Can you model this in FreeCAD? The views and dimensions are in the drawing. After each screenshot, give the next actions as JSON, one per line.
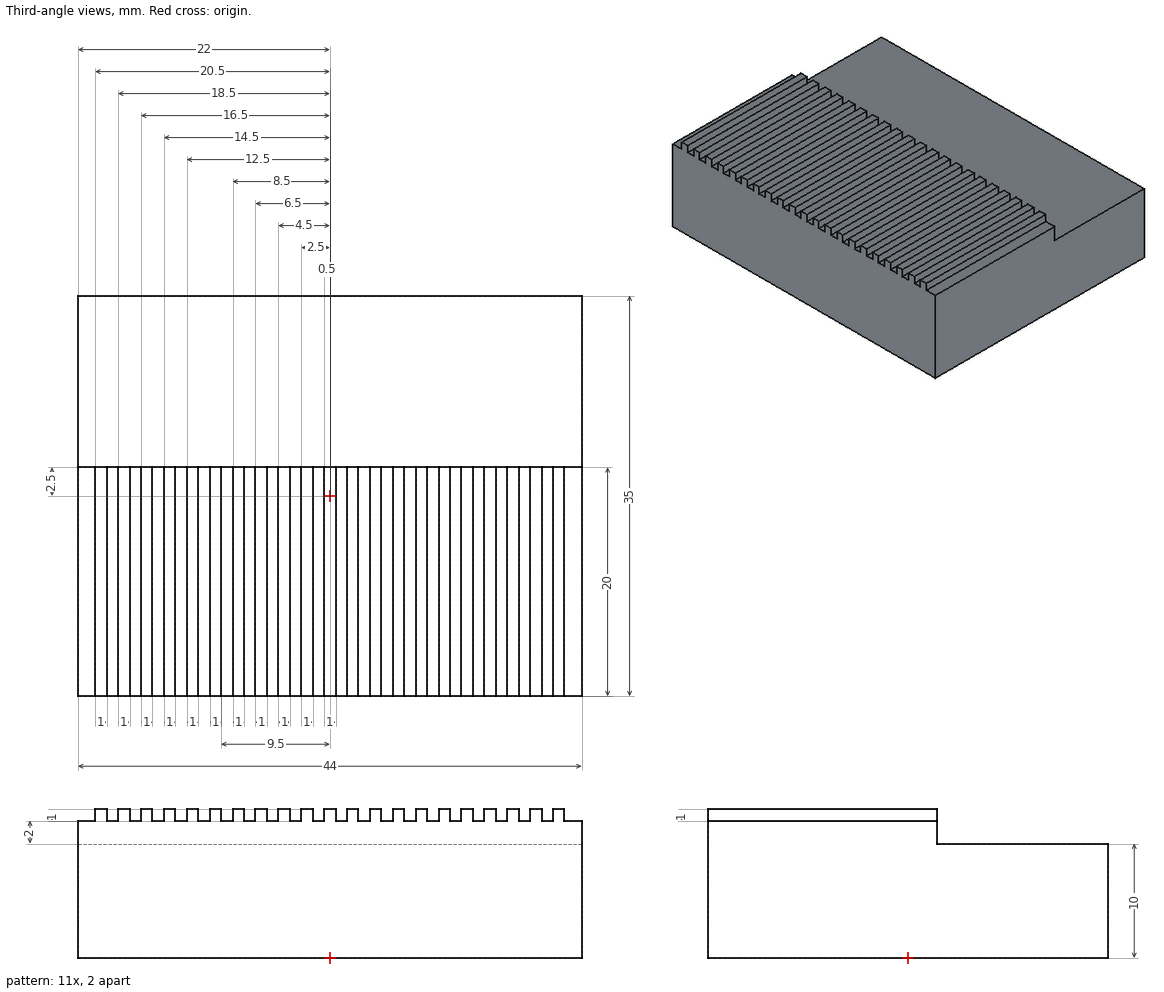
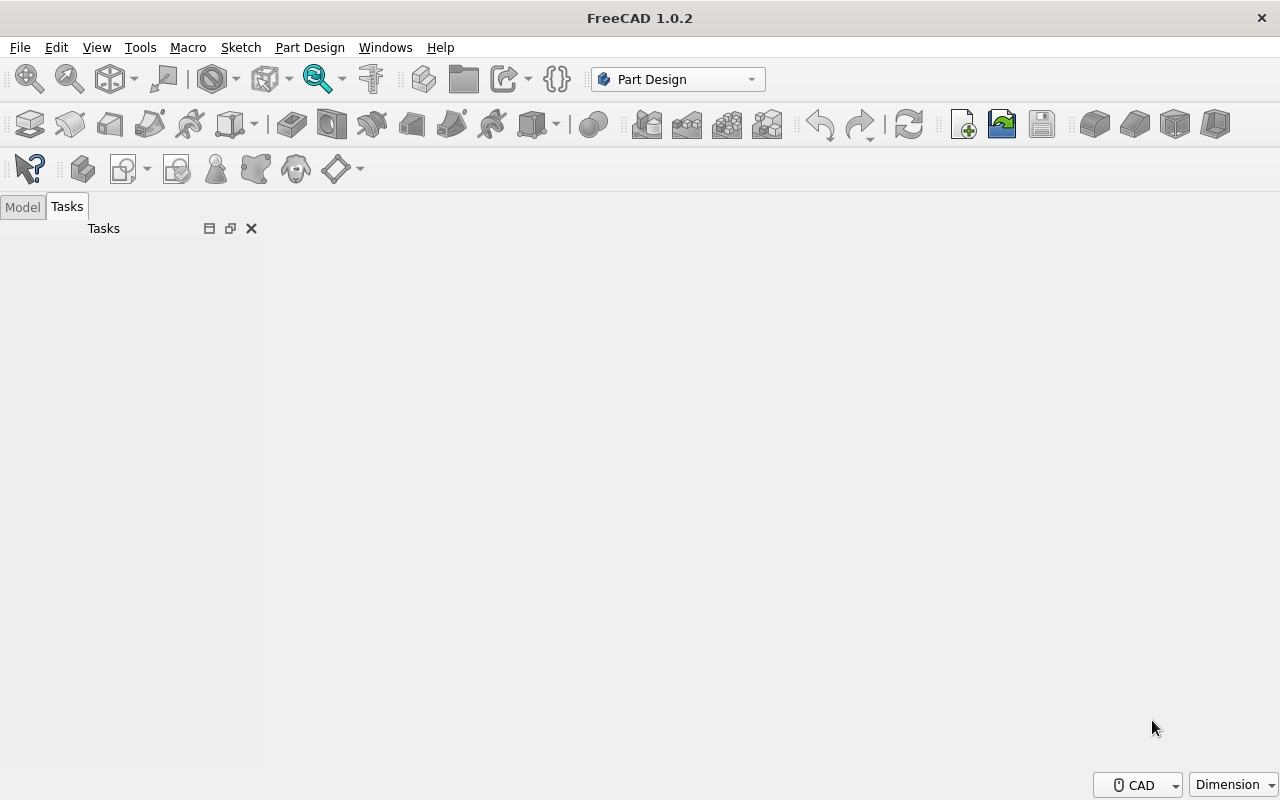
{"action": "left_click", "coordinate": [962, 124]}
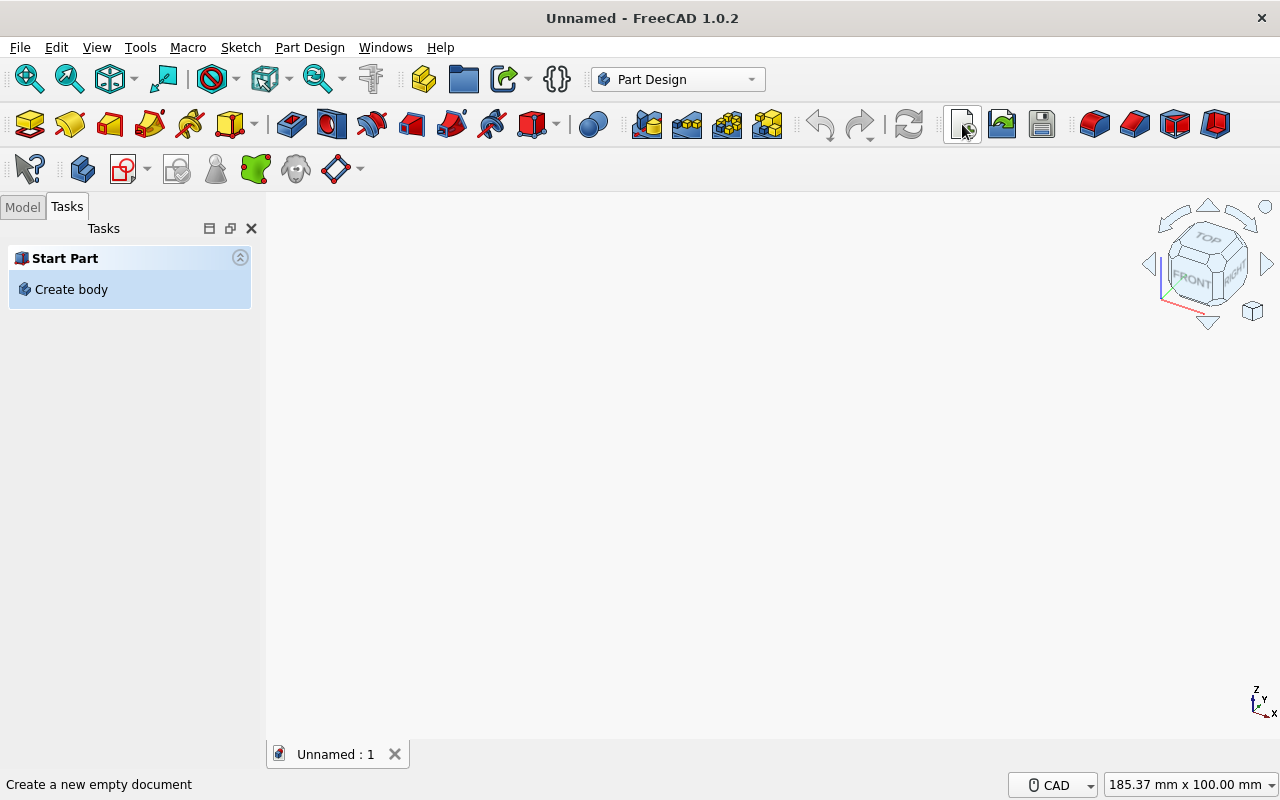
{"action": "left_click", "coordinate": [124, 170]}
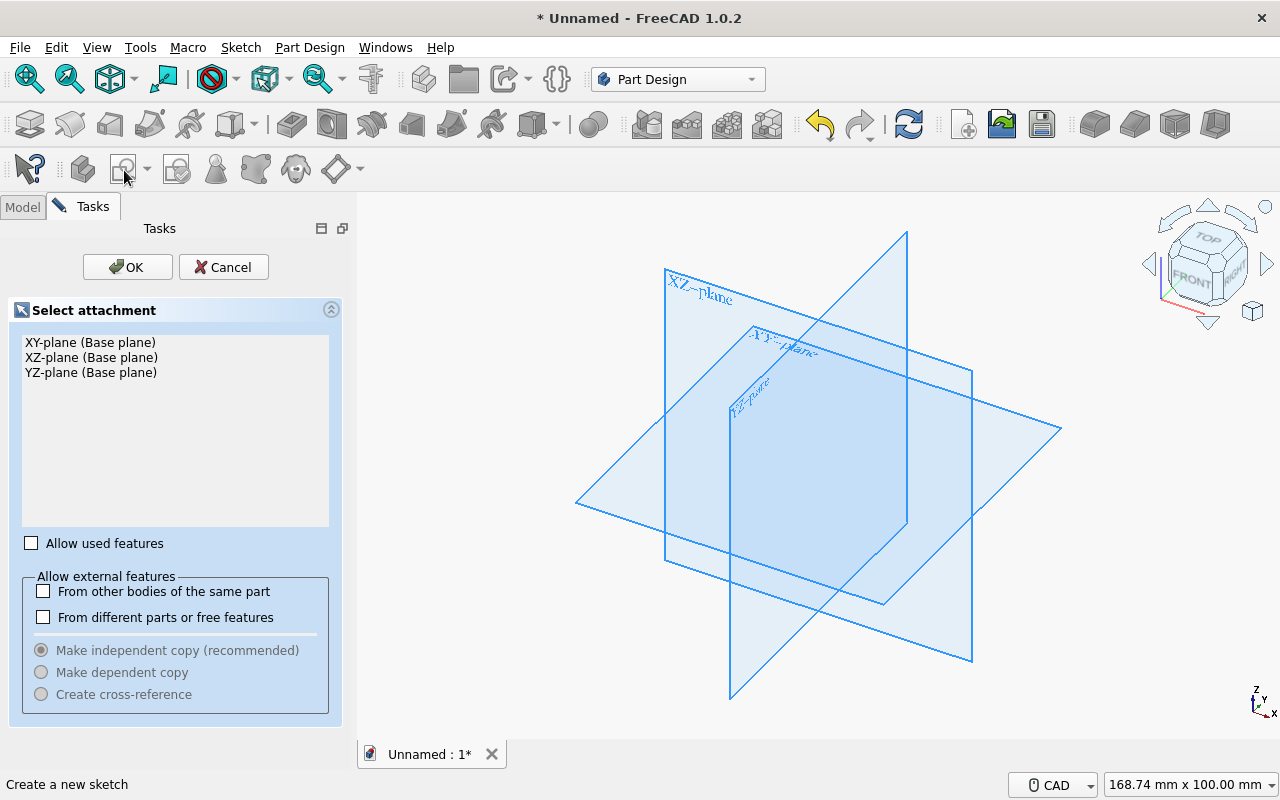
{"action": "left_click", "coordinate": [82, 342]}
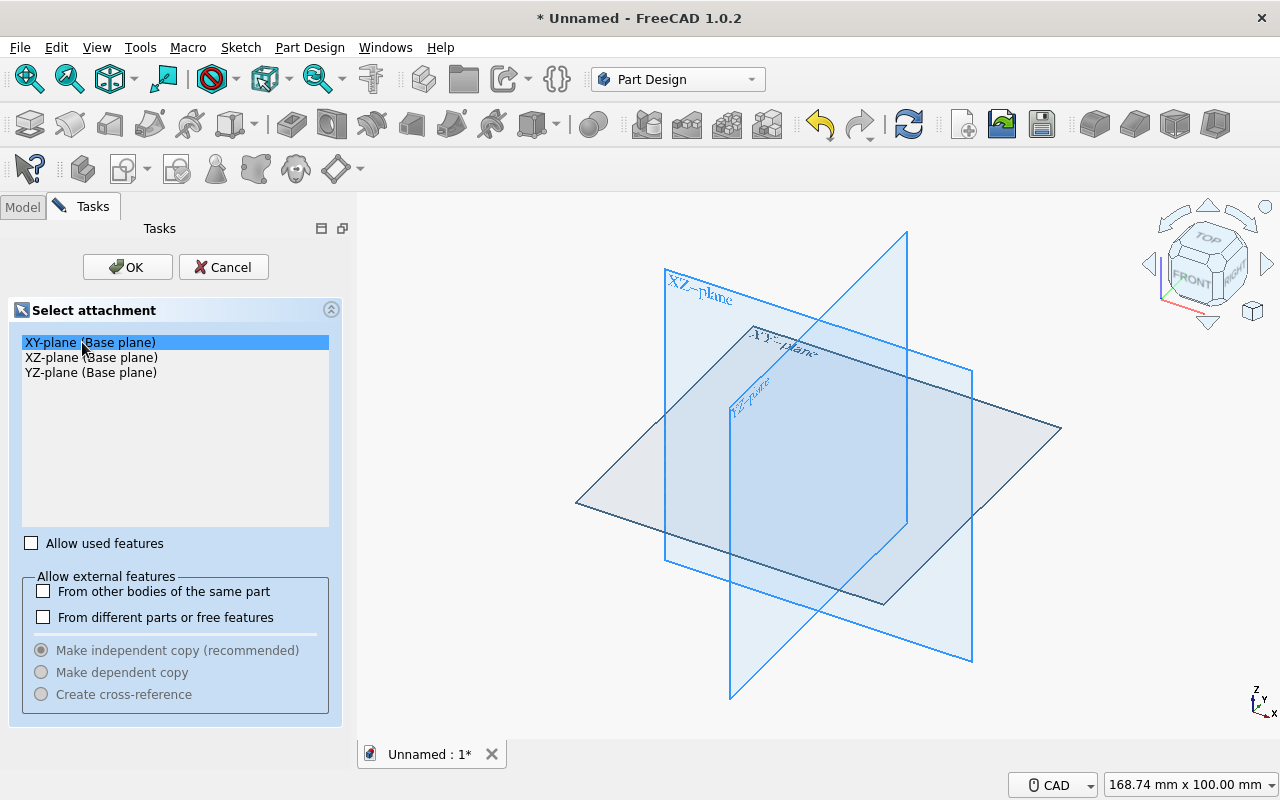
{"action": "left_click", "coordinate": [128, 267]}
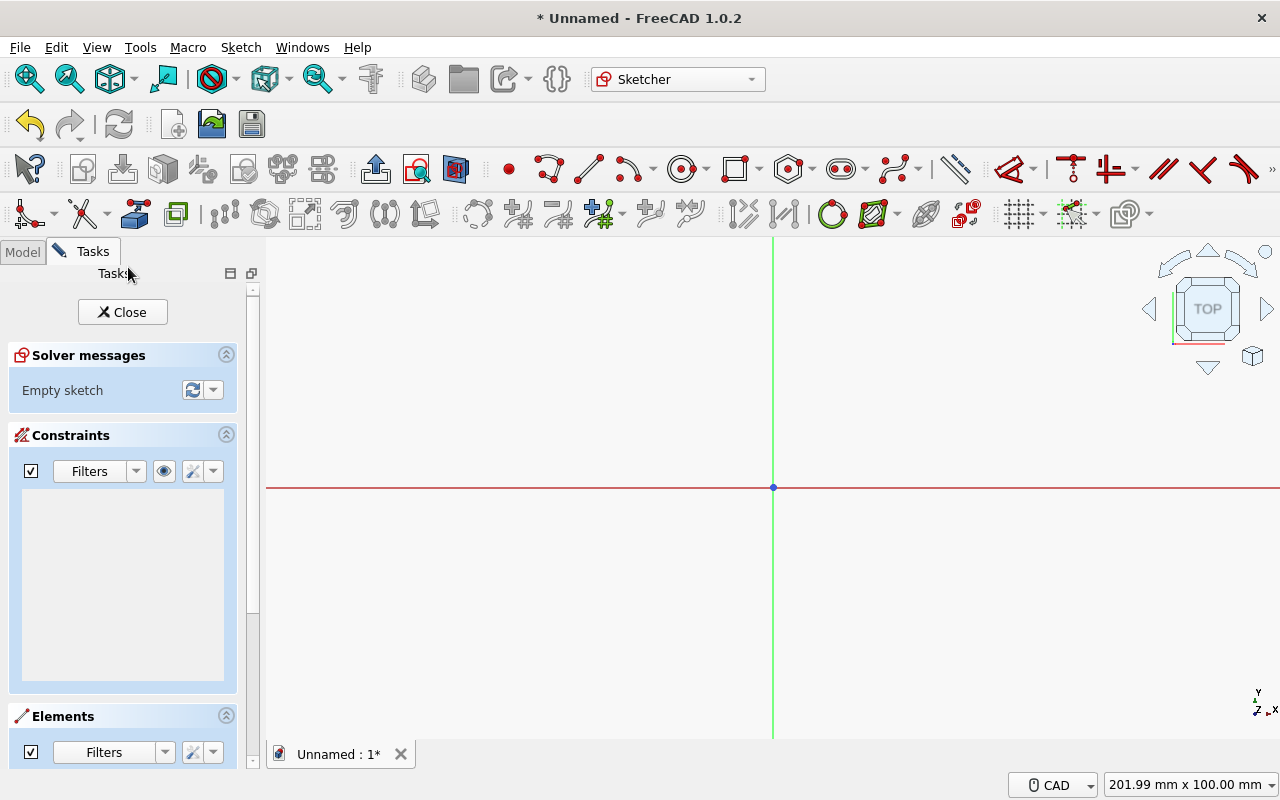
{"action": "scroll", "coordinate": [856, 488], "scroll_direction": "up", "scroll_amount": 3}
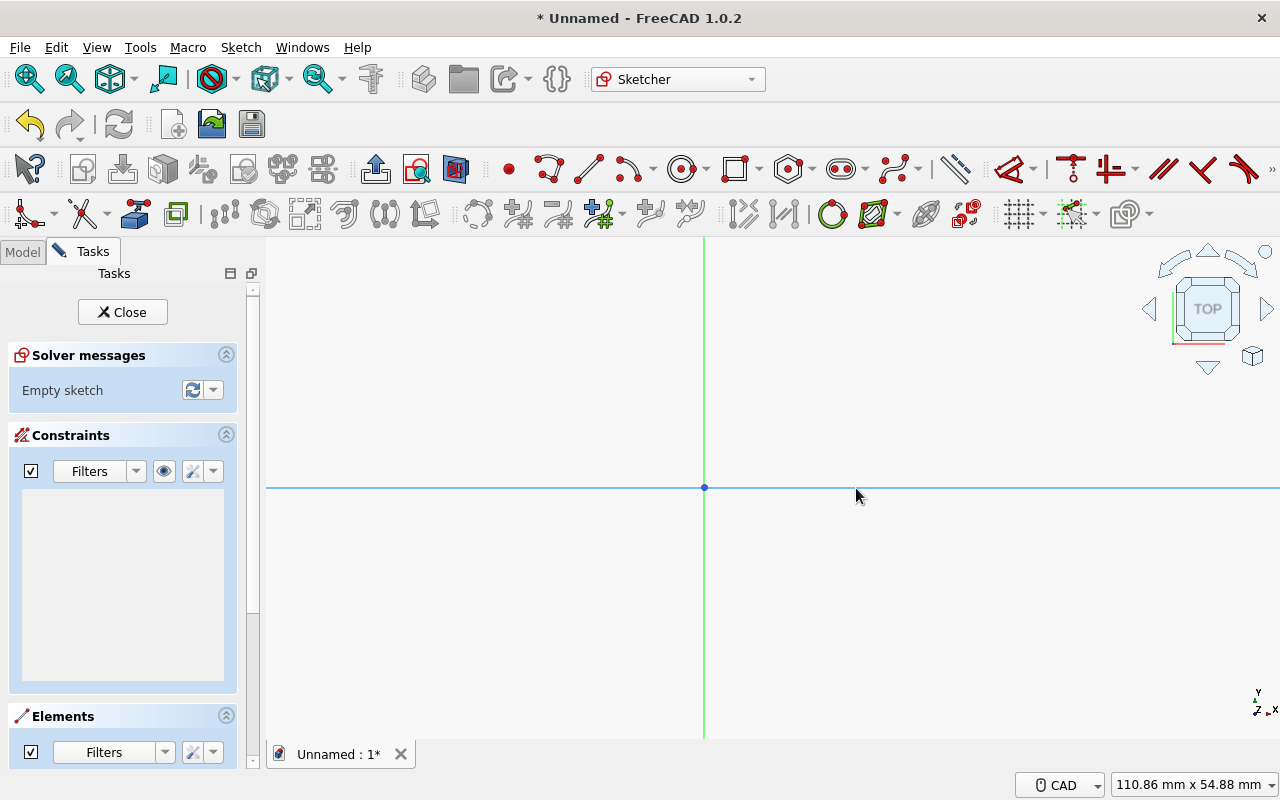
{"action": "left_click", "coordinate": [762, 170]}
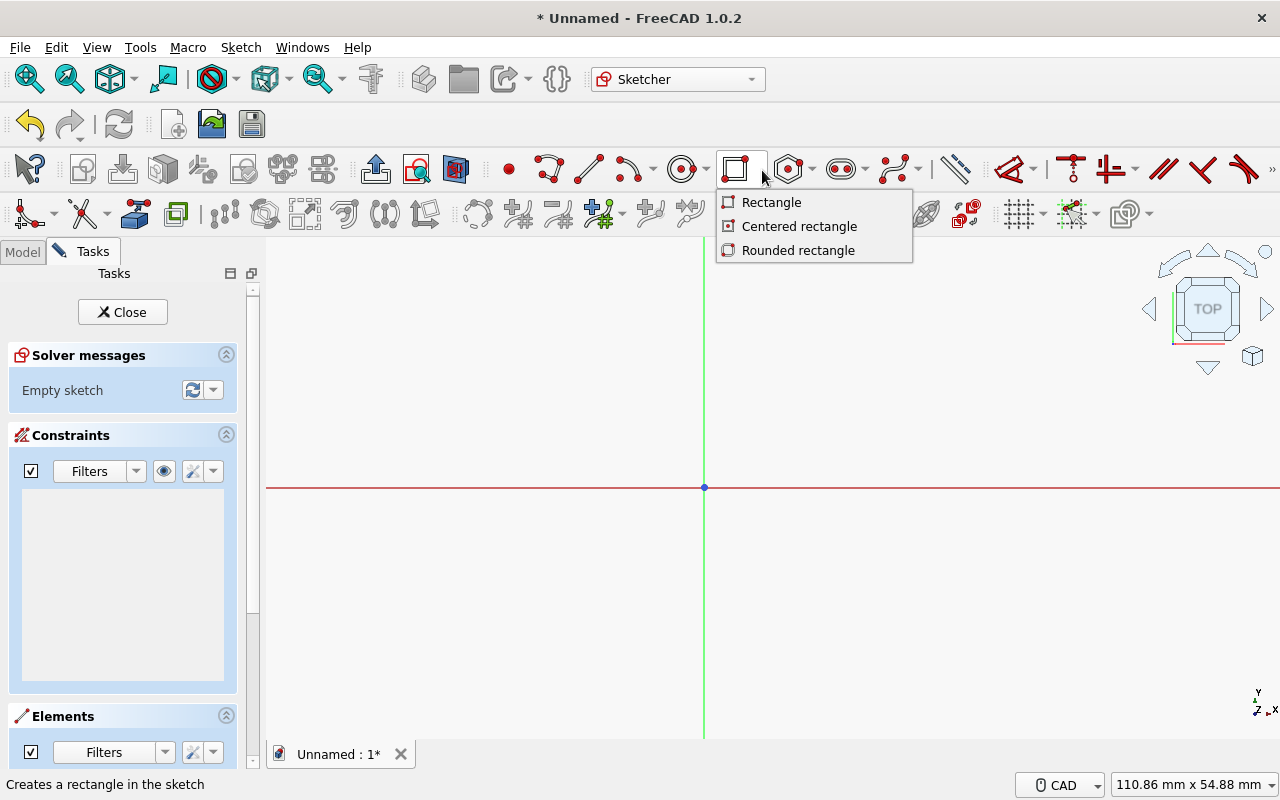
{"action": "left_click", "coordinate": [814, 226]}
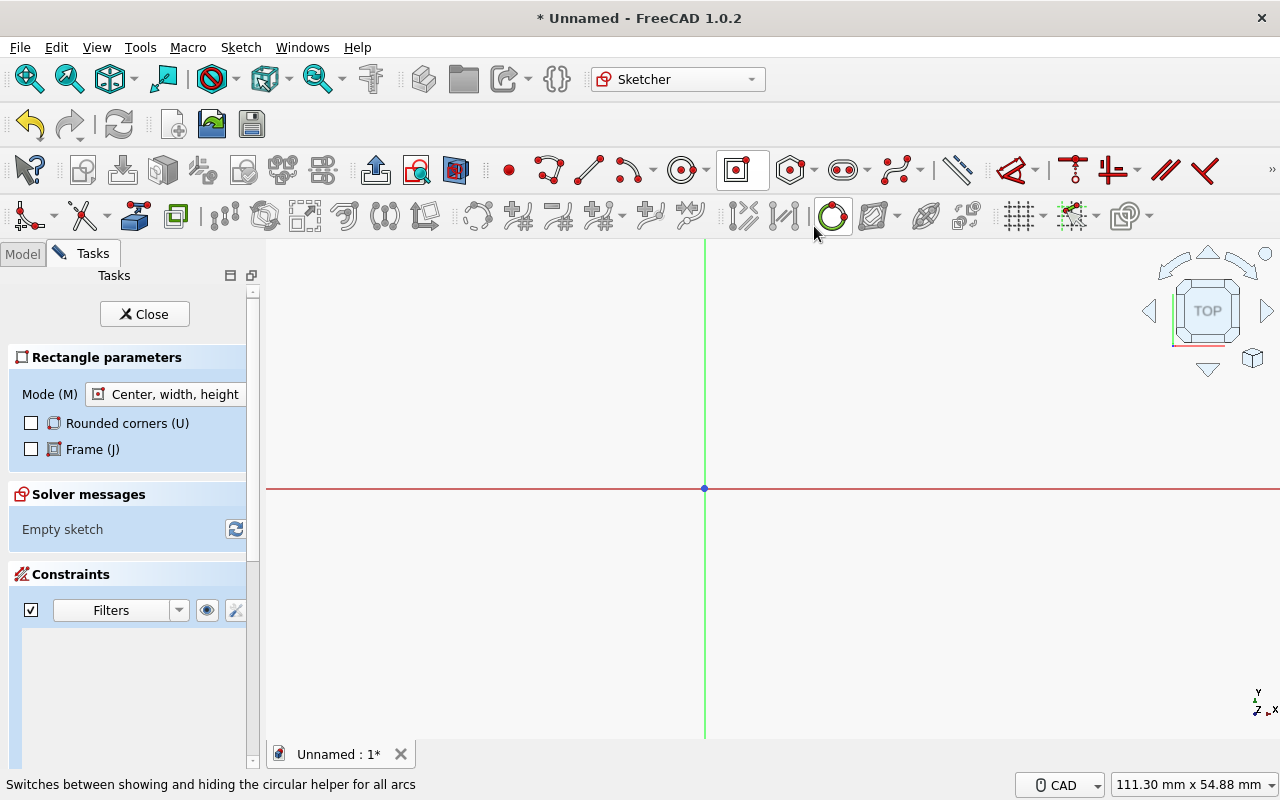
{"action": "left_click", "coordinate": [705, 489]}
{"action": "mouse_move", "coordinate": [905, 329]}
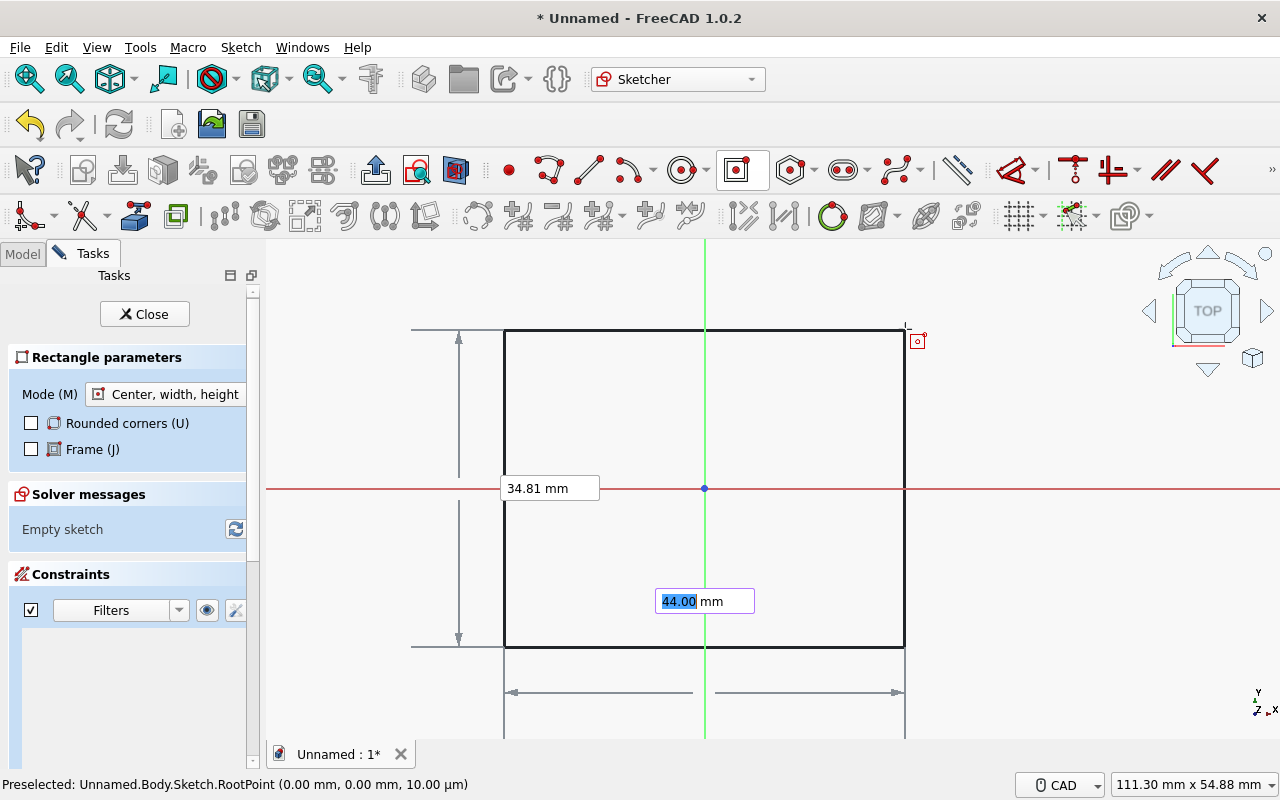
{"action": "type", "text": "44"}
{"action": "key", "text": "Tab"}
{"action": "type", "text": "35"}
{"action": "key", "text": "Return"}
{"action": "key", "text": "Escape"}